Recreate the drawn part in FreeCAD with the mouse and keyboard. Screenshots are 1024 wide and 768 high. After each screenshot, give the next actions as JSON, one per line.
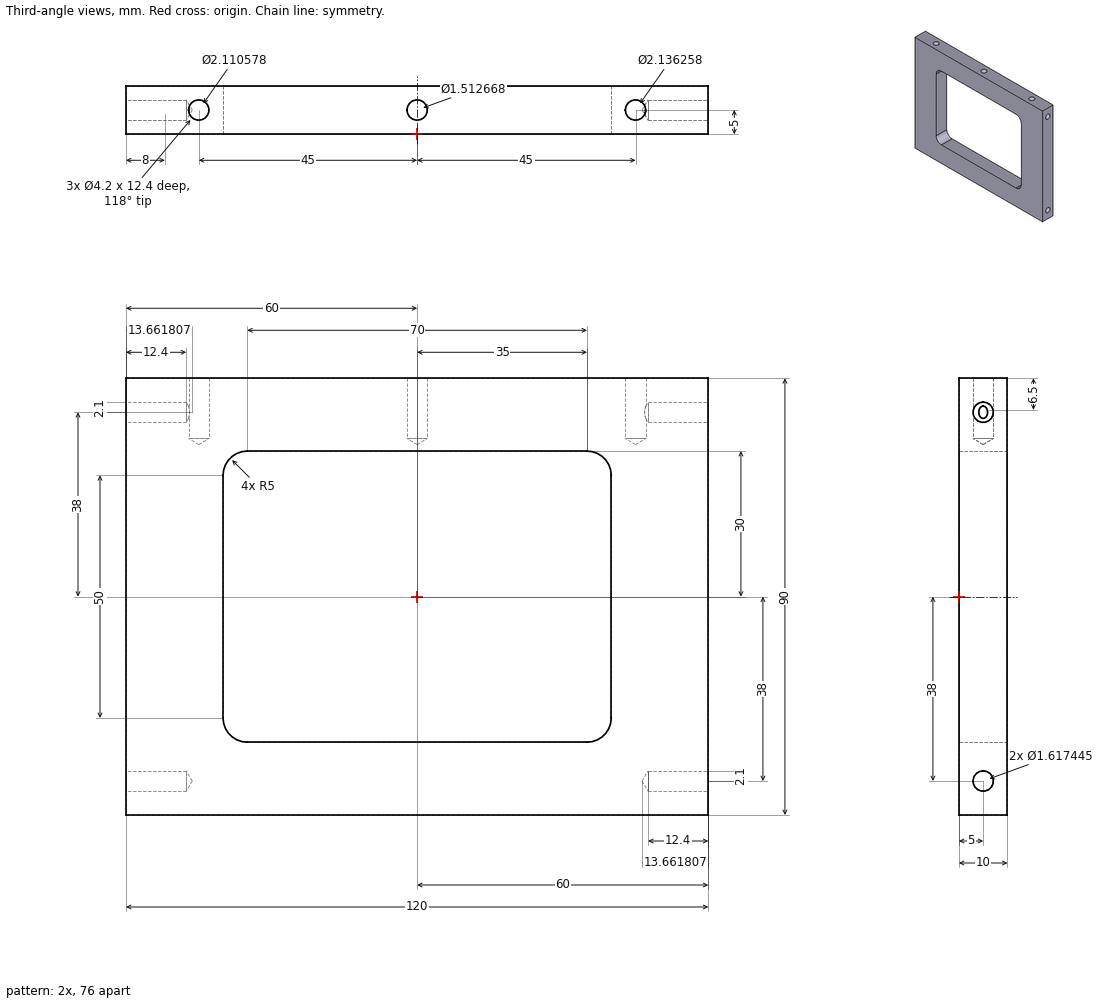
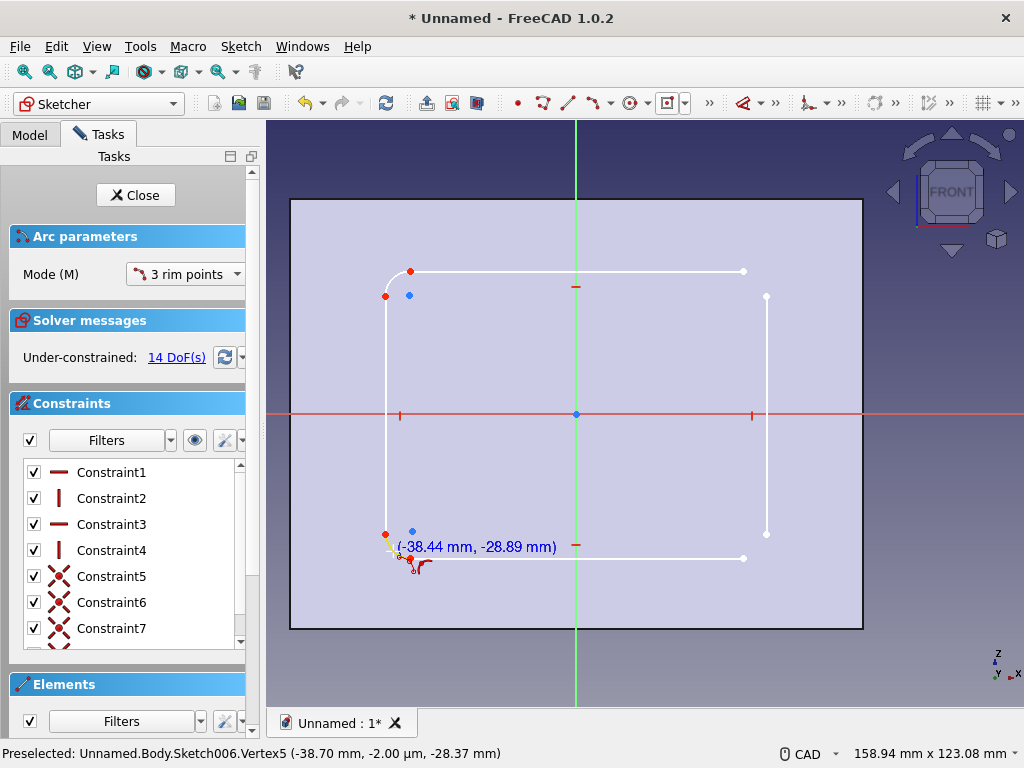
{"action": "left_click", "coordinate": [743, 559]}
{"action": "left_click", "coordinate": [767, 534]}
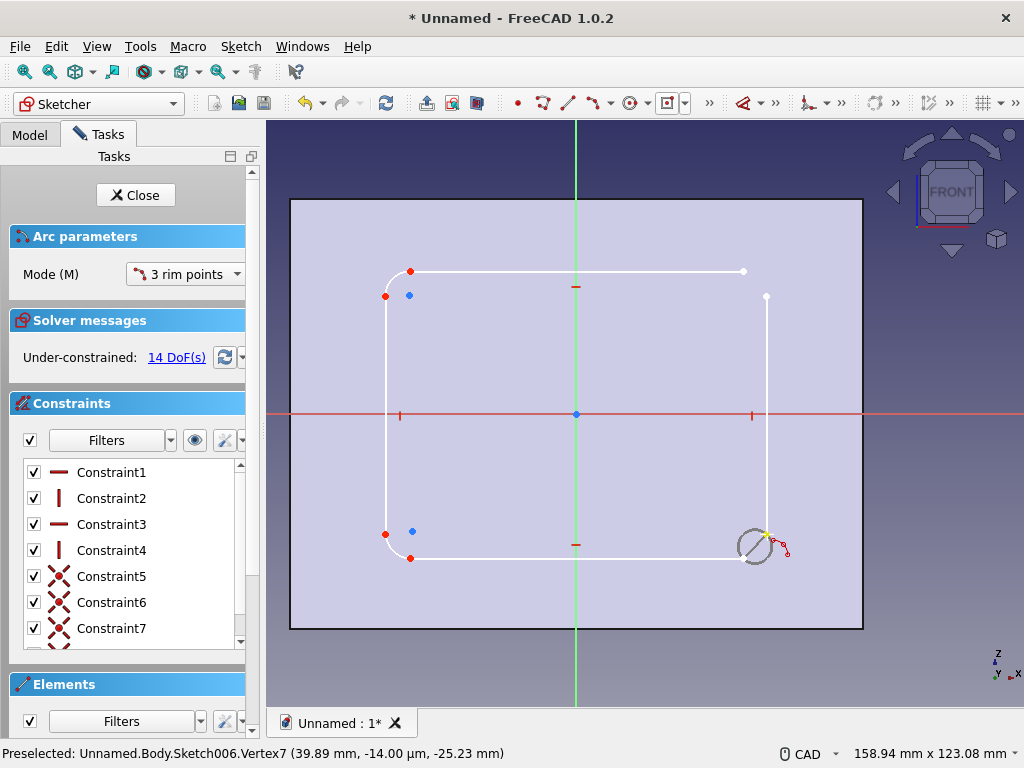
{"action": "scroll", "coordinate": [760, 550], "scroll_direction": "up", "scroll_amount": 5}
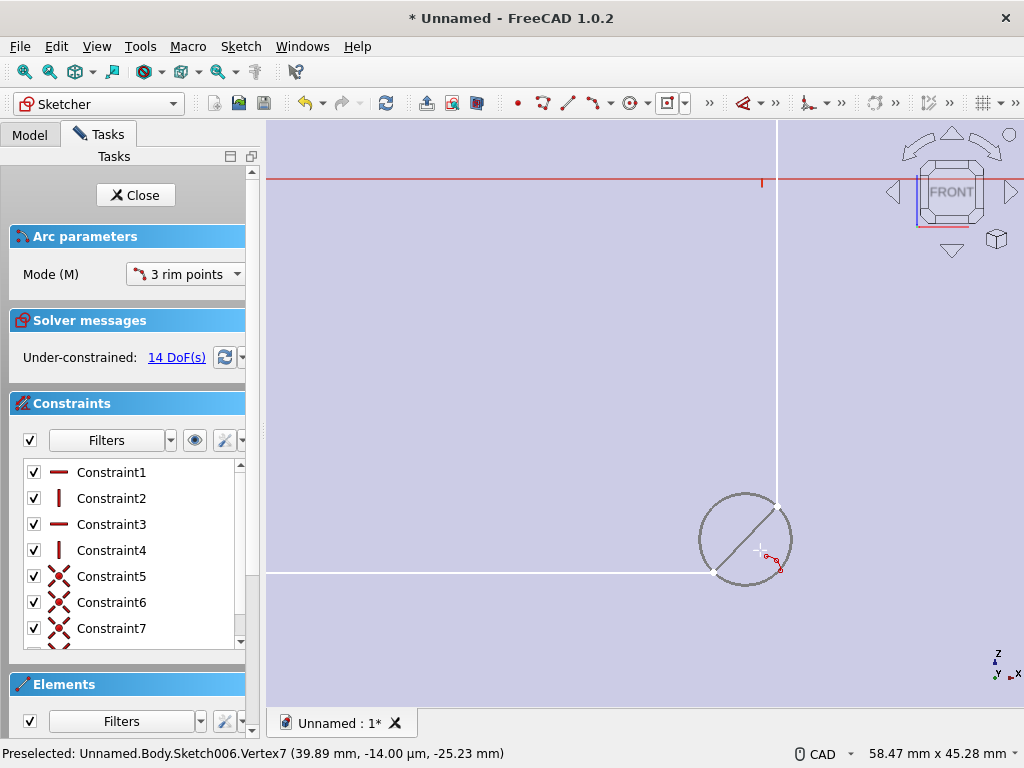
{"action": "left_click", "coordinate": [759, 549]}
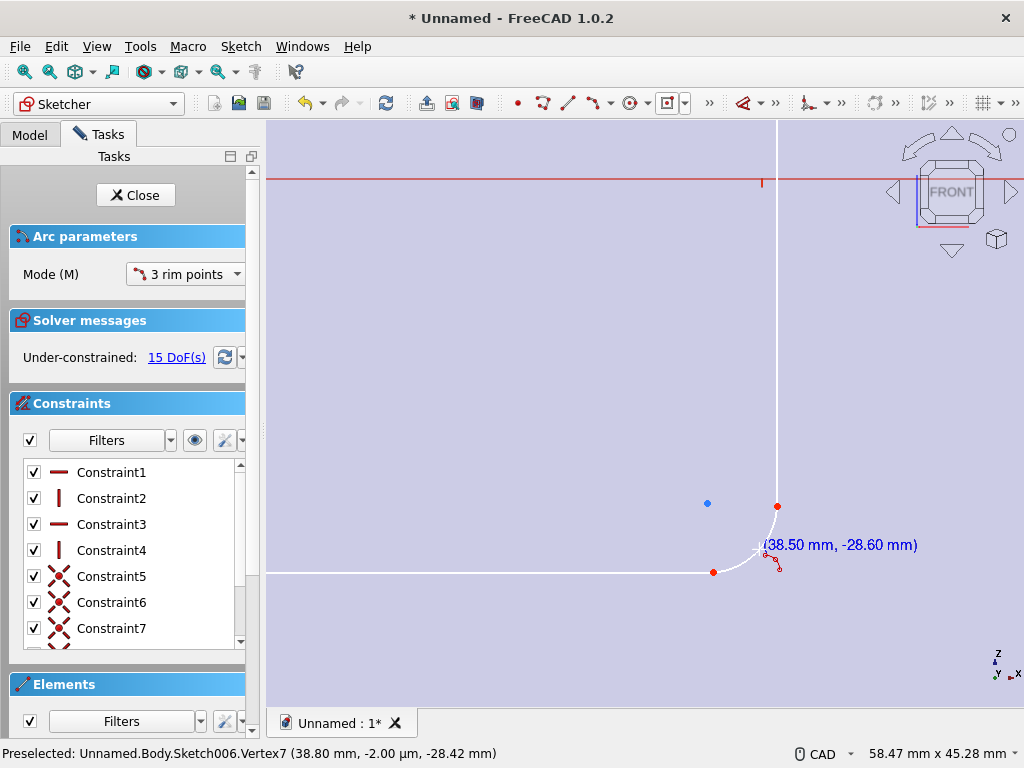
{"action": "scroll", "coordinate": [761, 550], "scroll_direction": "down", "scroll_amount": 5}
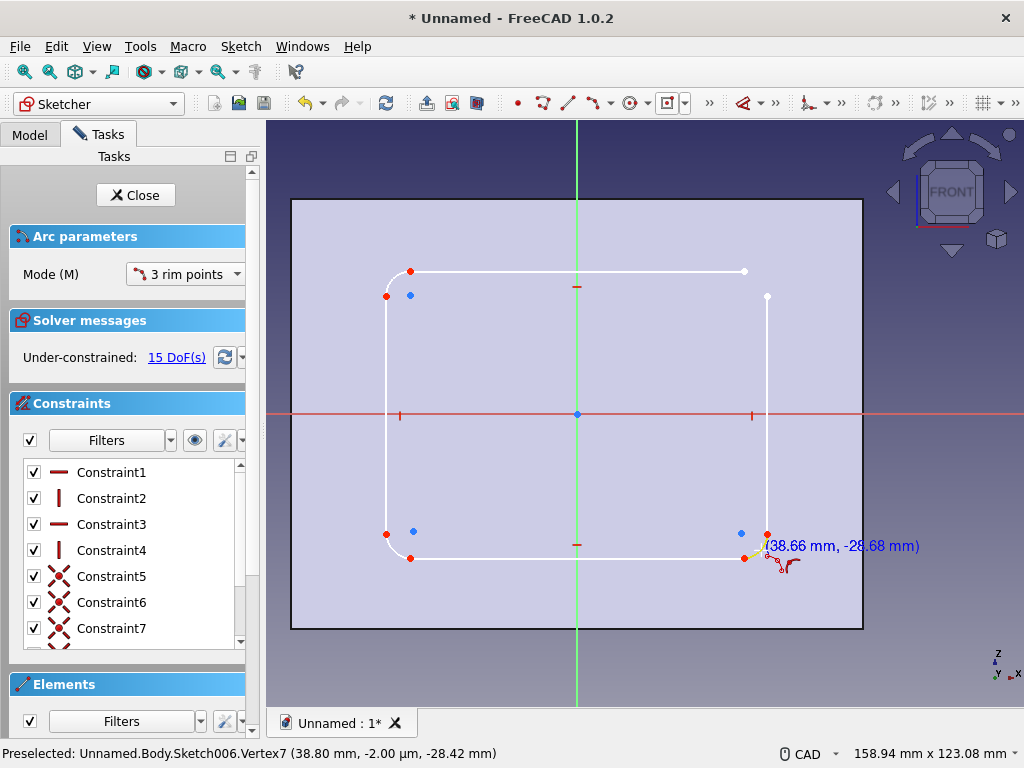
{"action": "left_click", "coordinate": [767, 296]}
{"action": "left_click", "coordinate": [744, 272]}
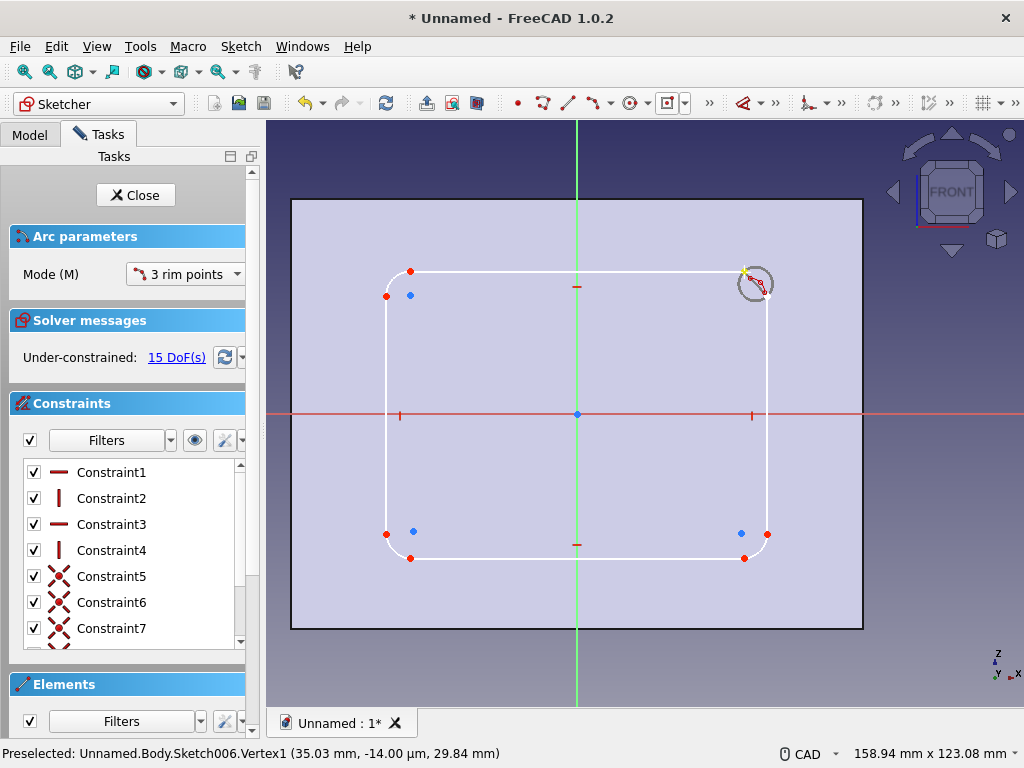
{"action": "scroll", "coordinate": [761, 278], "scroll_direction": "up", "scroll_amount": 5}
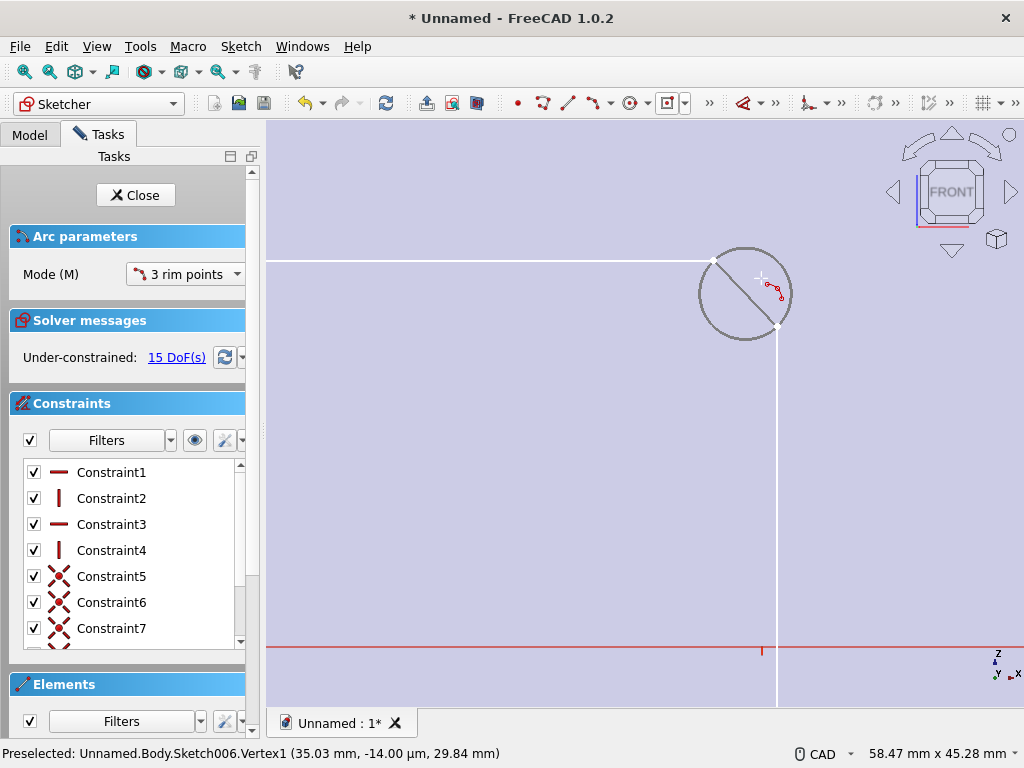
{"action": "left_click", "coordinate": [759, 277]}
{"action": "key", "text": "Escape"}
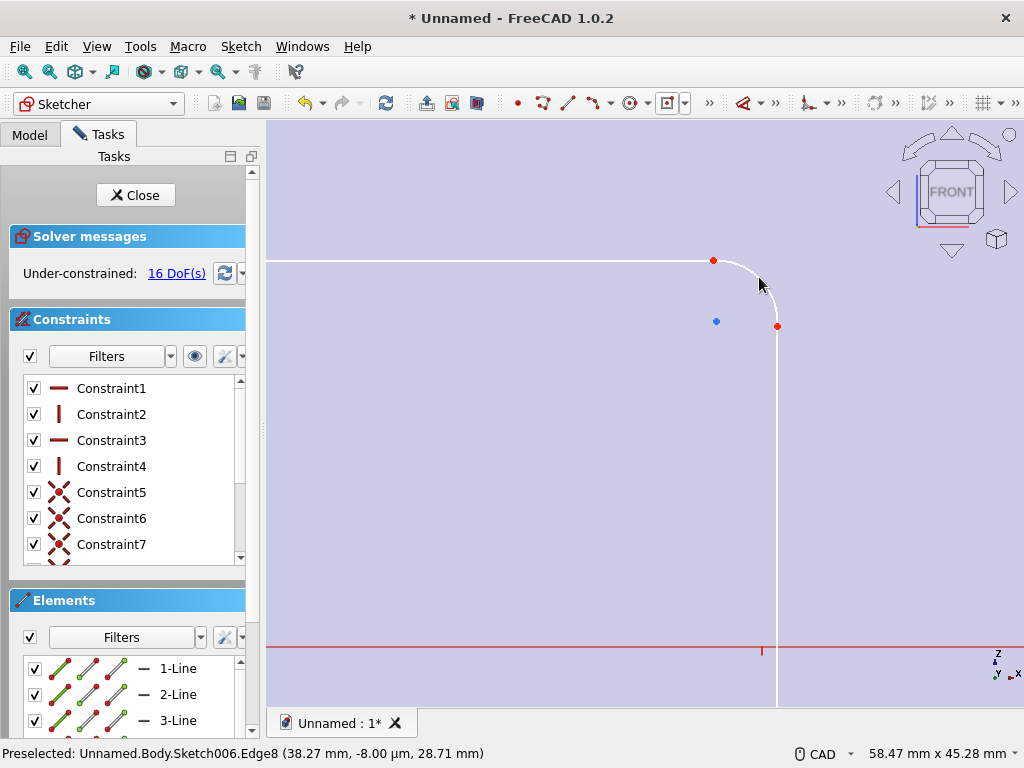
{"action": "left_click", "coordinate": [442, 261]}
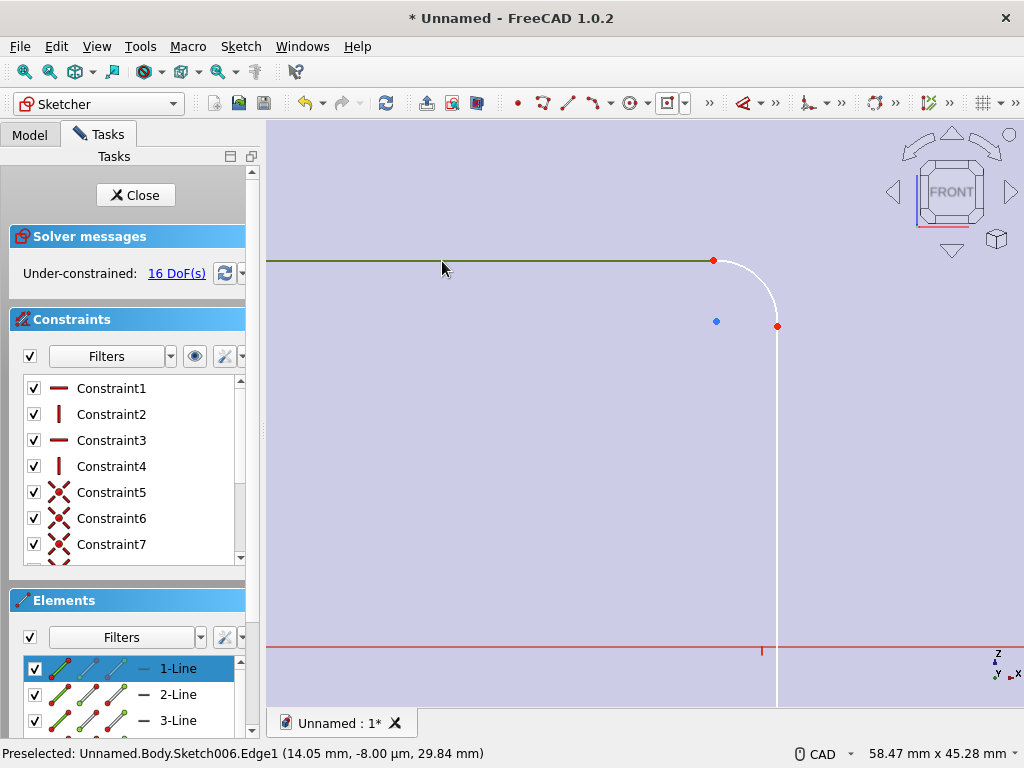
{"action": "scroll", "coordinate": [761, 277], "scroll_direction": "down", "scroll_amount": 5}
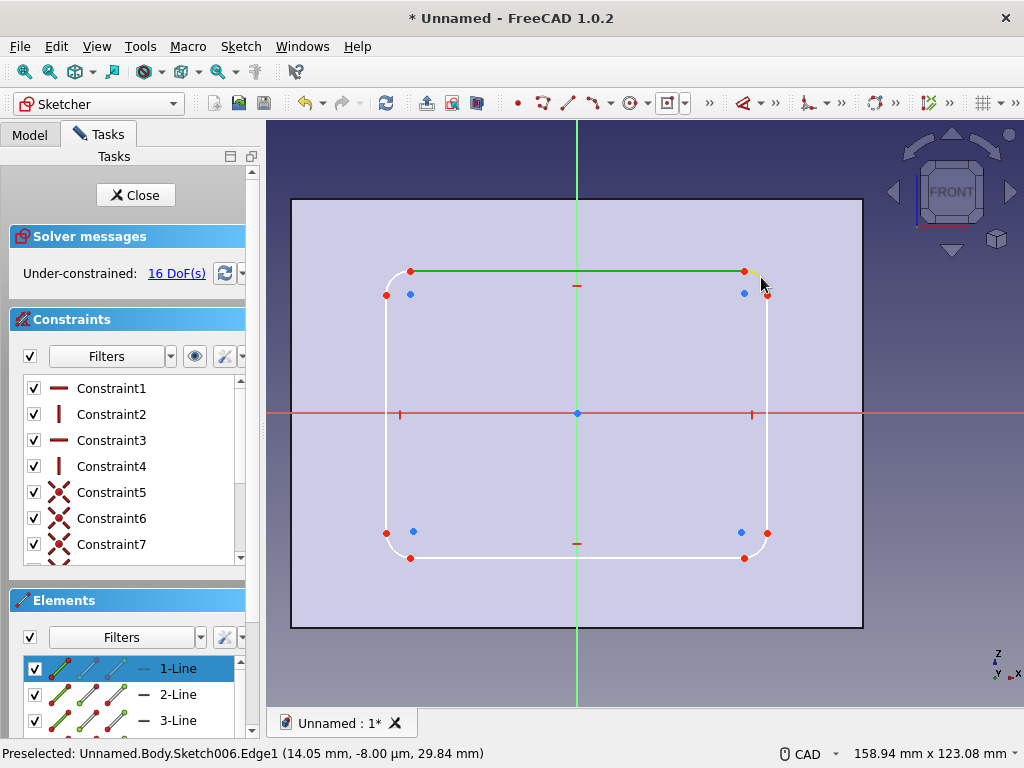
{"action": "left_click", "coordinate": [399, 274]}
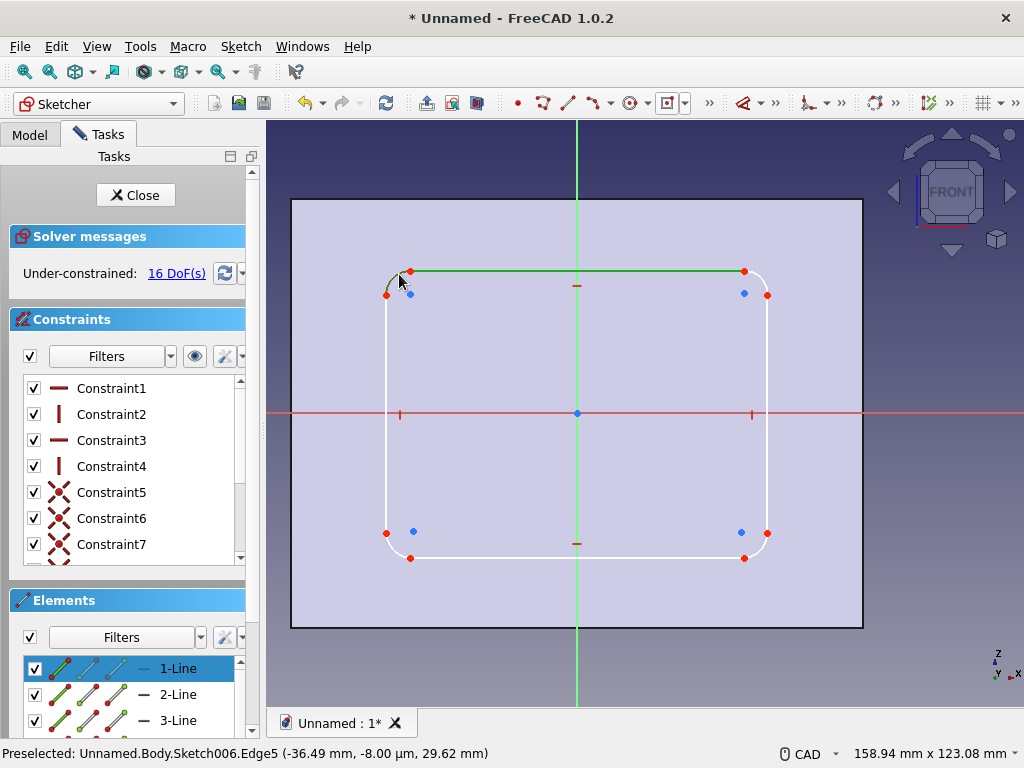
{"action": "key", "text": "t"}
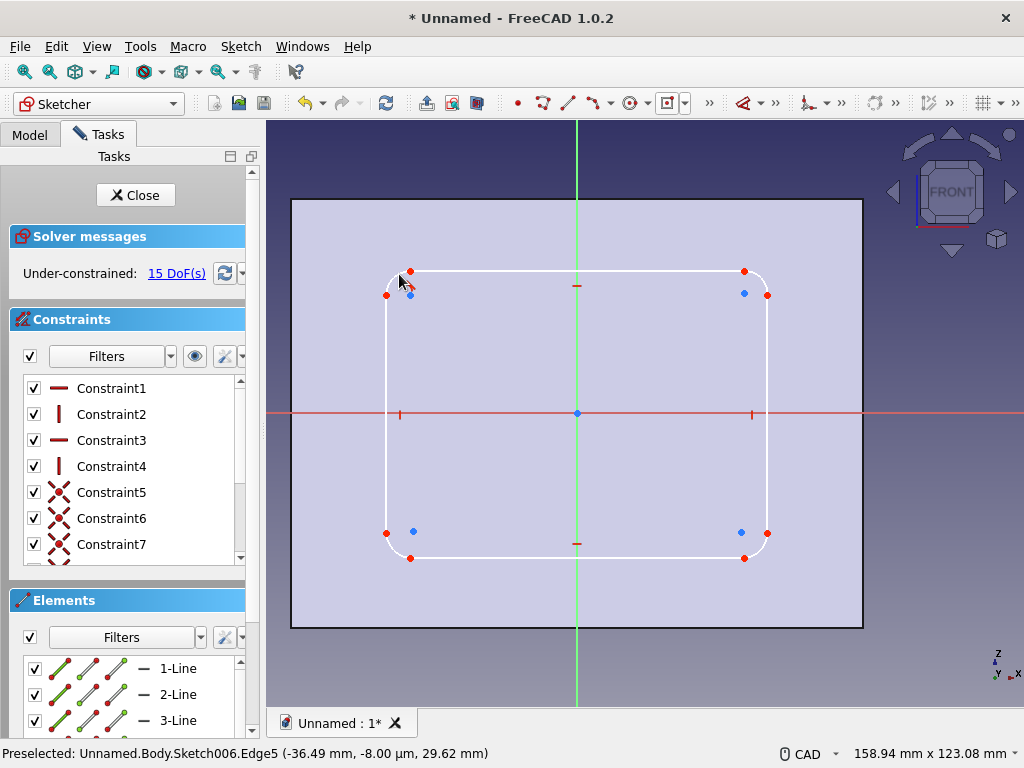
{"action": "left_click", "coordinate": [644, 271]}